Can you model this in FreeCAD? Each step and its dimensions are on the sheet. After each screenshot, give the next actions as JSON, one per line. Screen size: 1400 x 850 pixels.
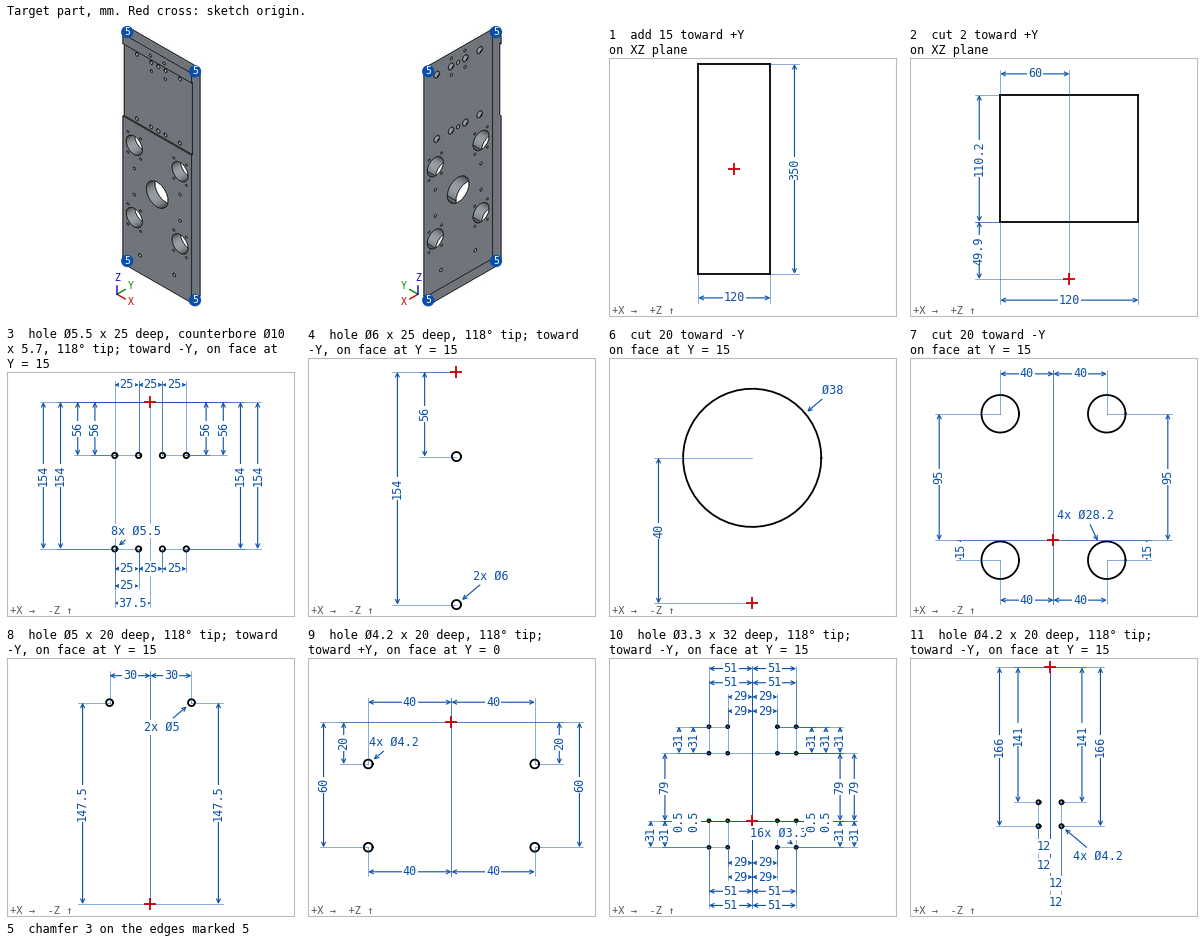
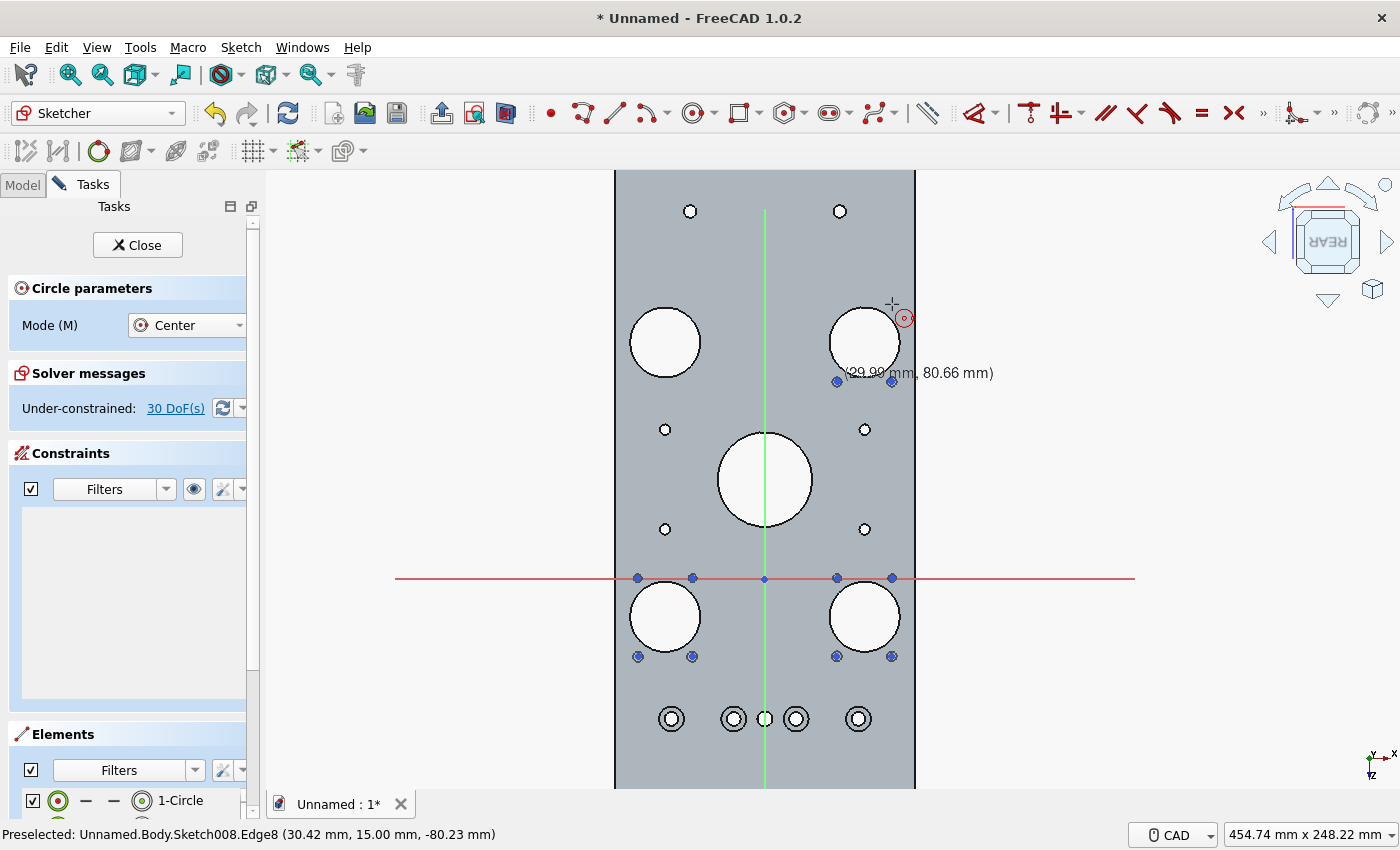
{"action": "left_click", "coordinate": [892, 304]}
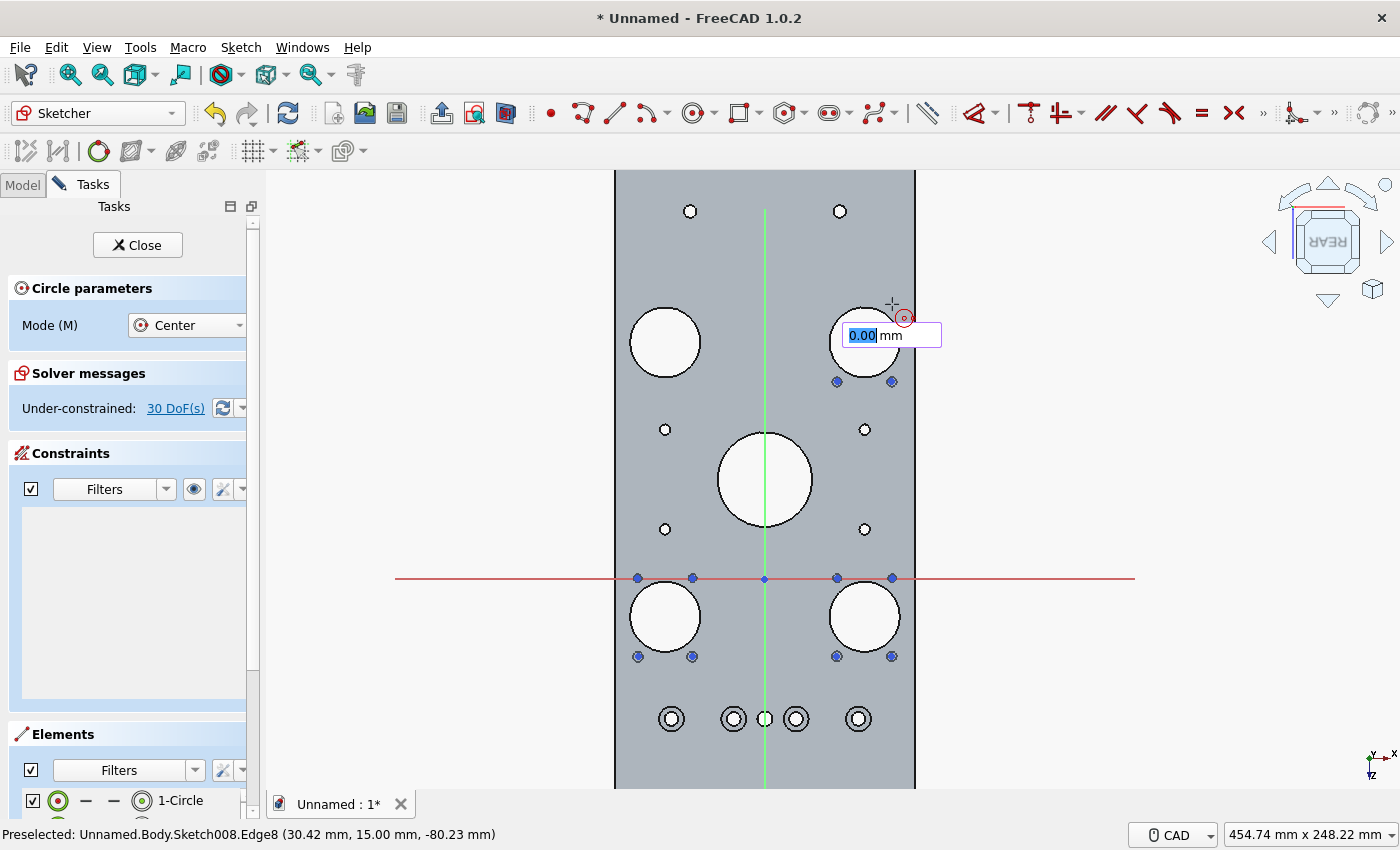
{"action": "scroll", "coordinate": [895, 301], "scroll_direction": "up", "scroll_amount": 7}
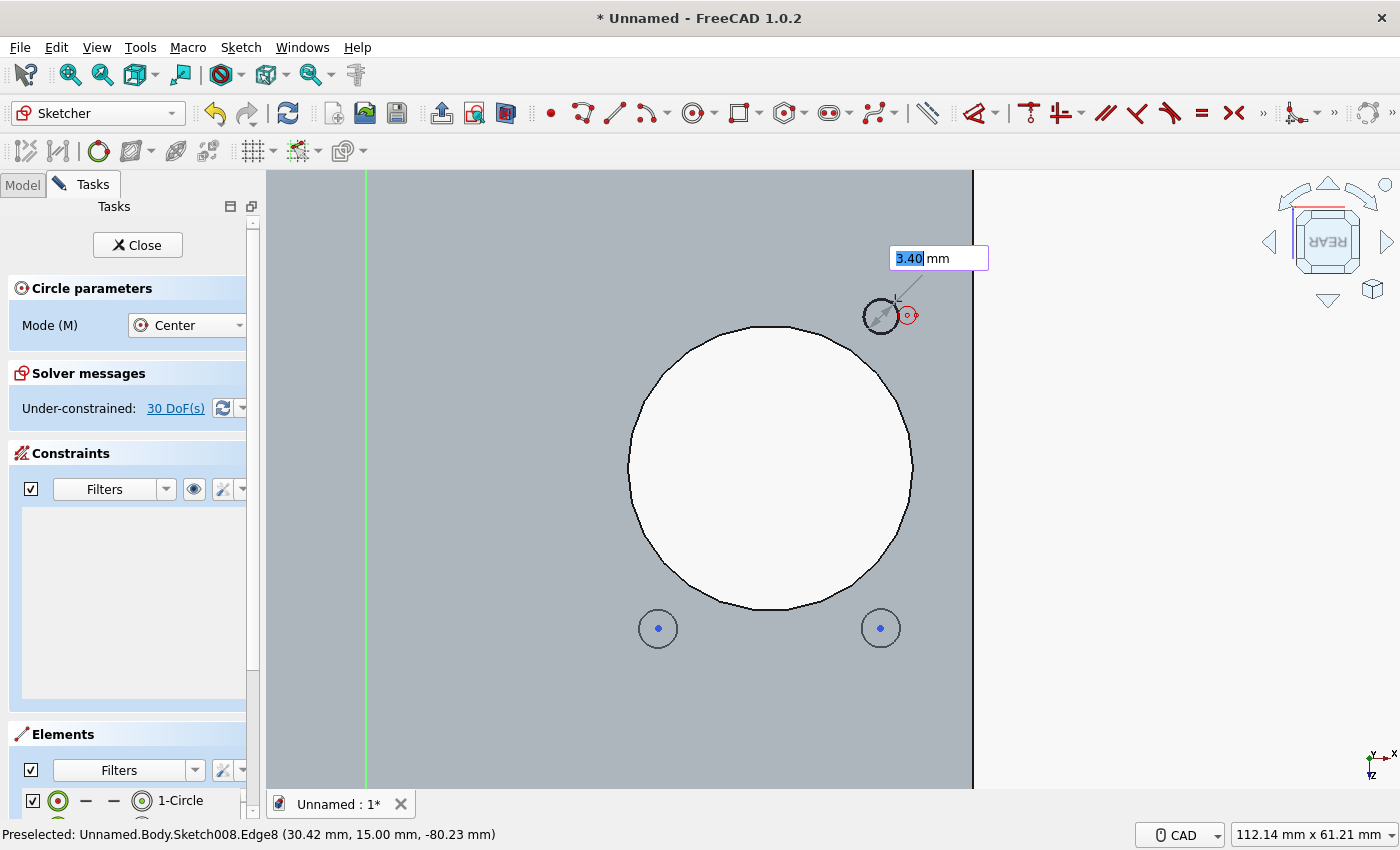
{"action": "left_click", "coordinate": [893, 300]}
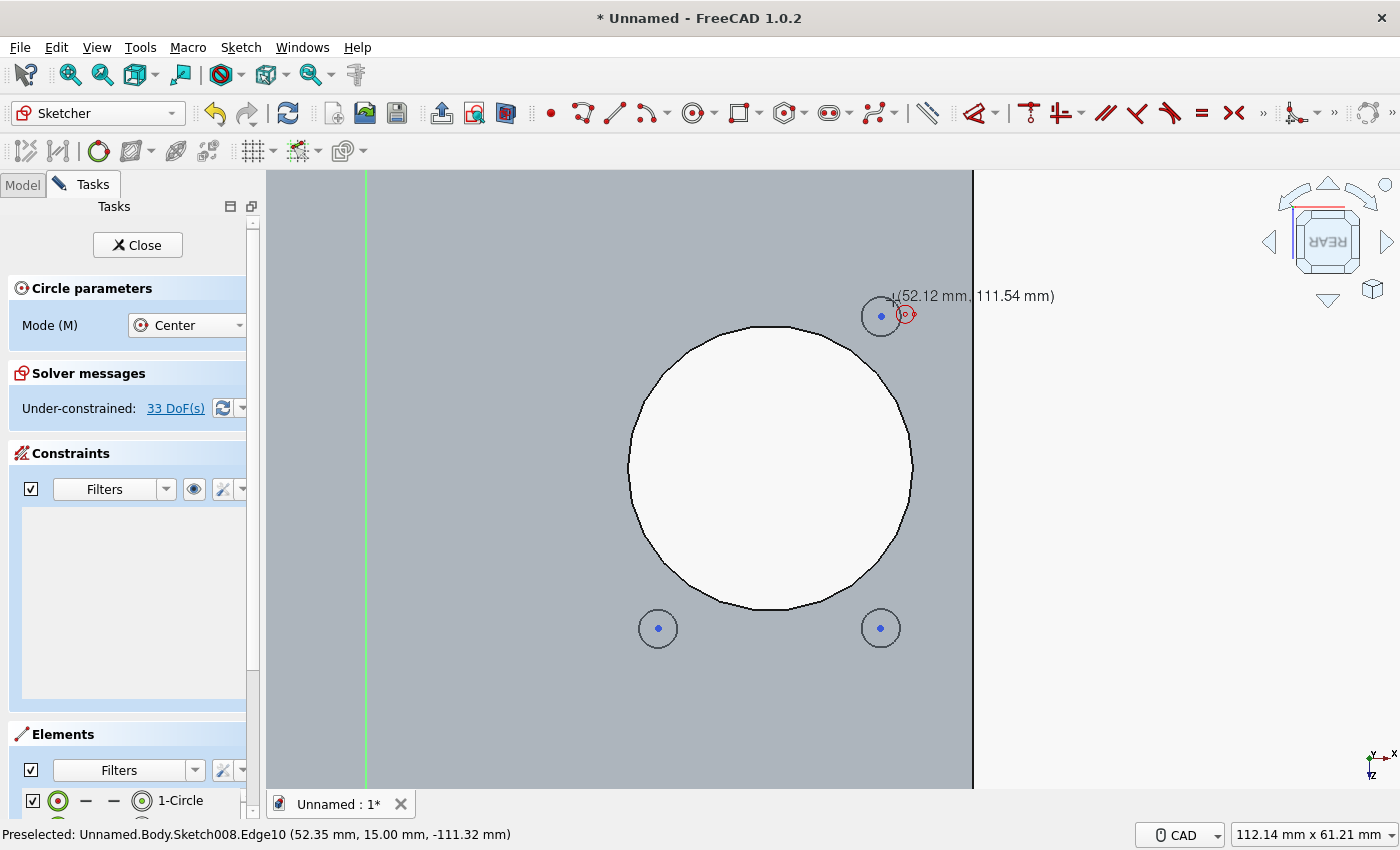
{"action": "scroll", "coordinate": [659, 312], "scroll_direction": "up", "scroll_amount": 2}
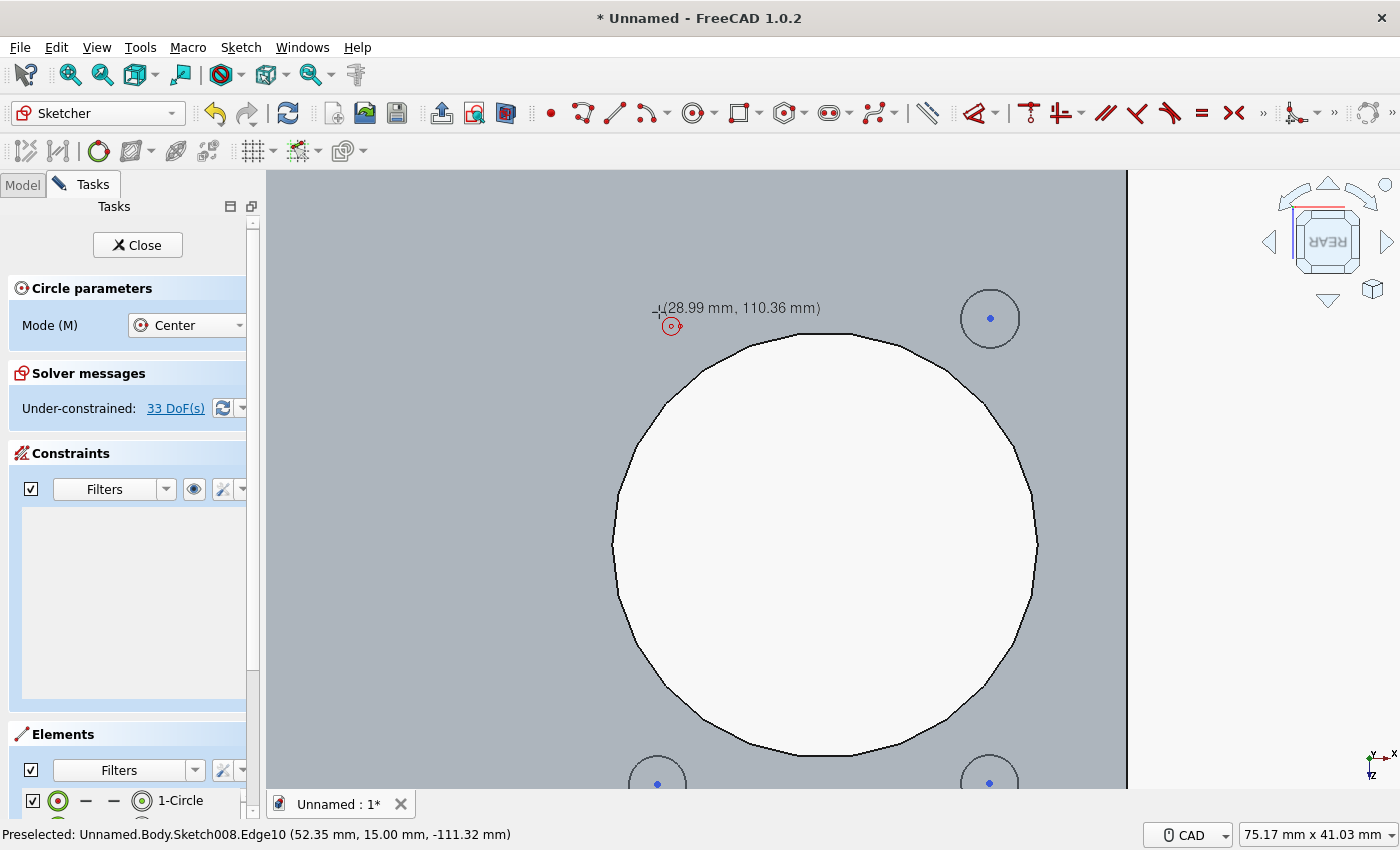
{"action": "scroll", "coordinate": [872, 302], "scroll_direction": "down", "scroll_amount": 9}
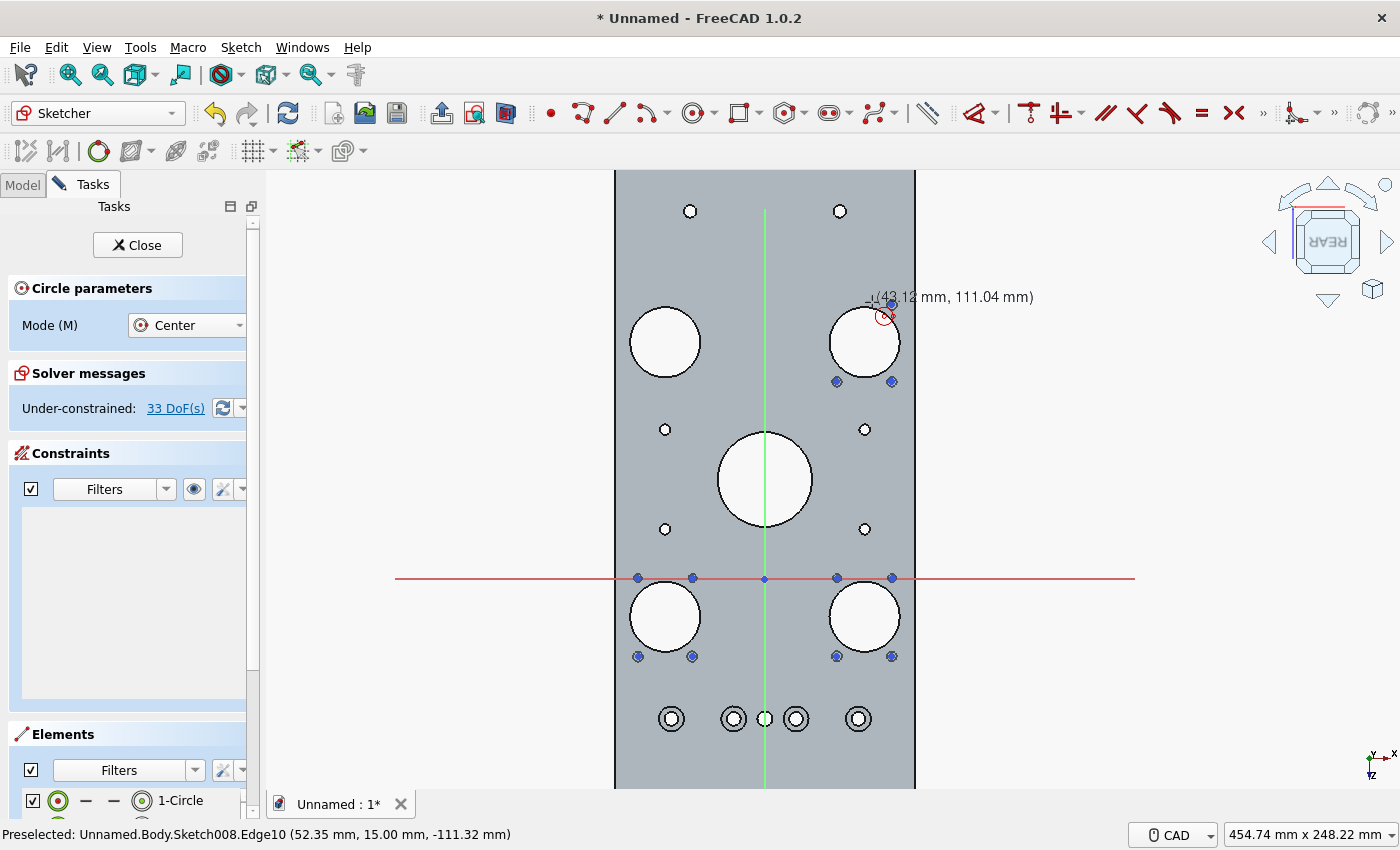
{"action": "left_click", "coordinate": [837, 304]}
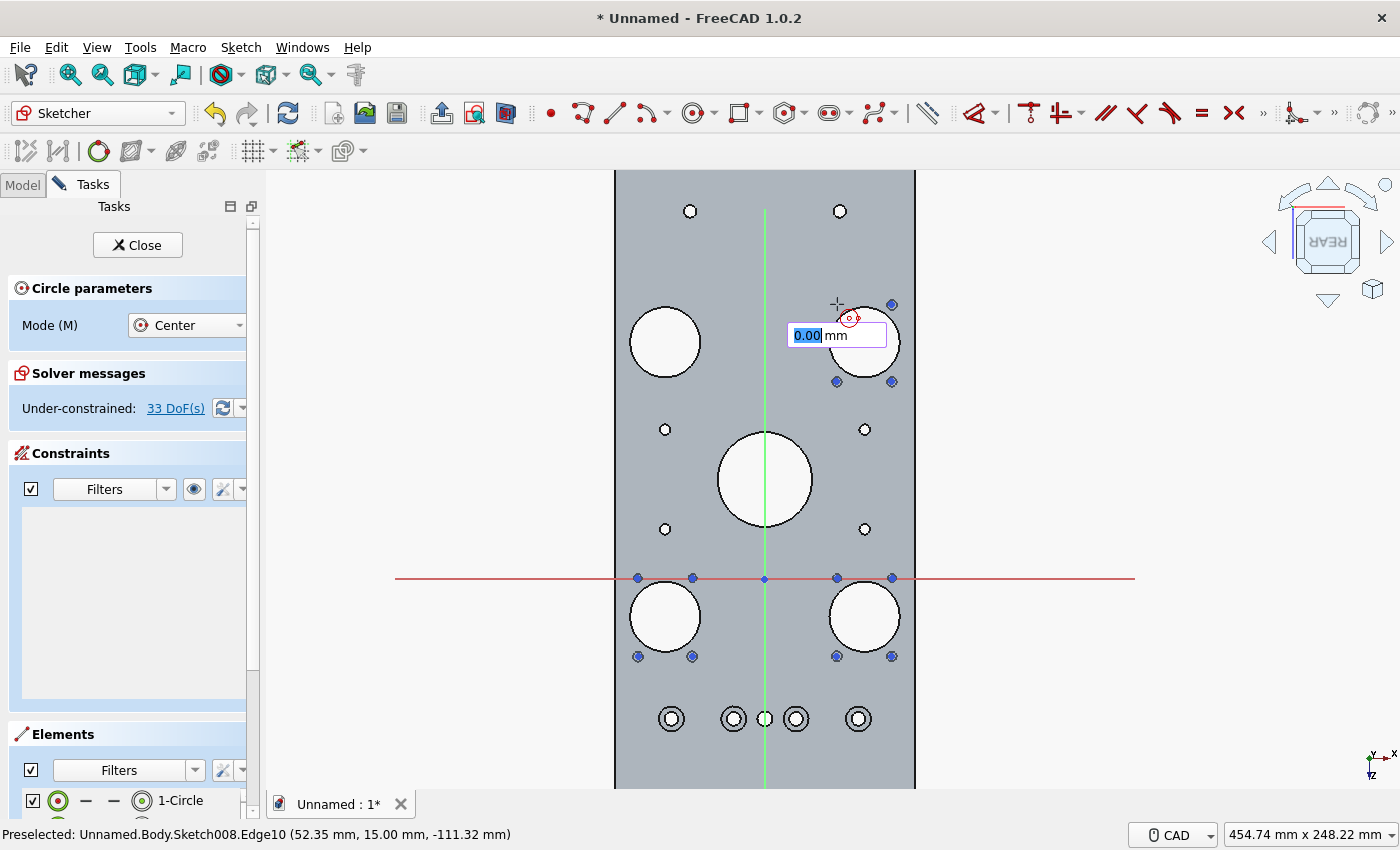
{"action": "scroll", "coordinate": [840, 301], "scroll_direction": "up", "scroll_amount": 7}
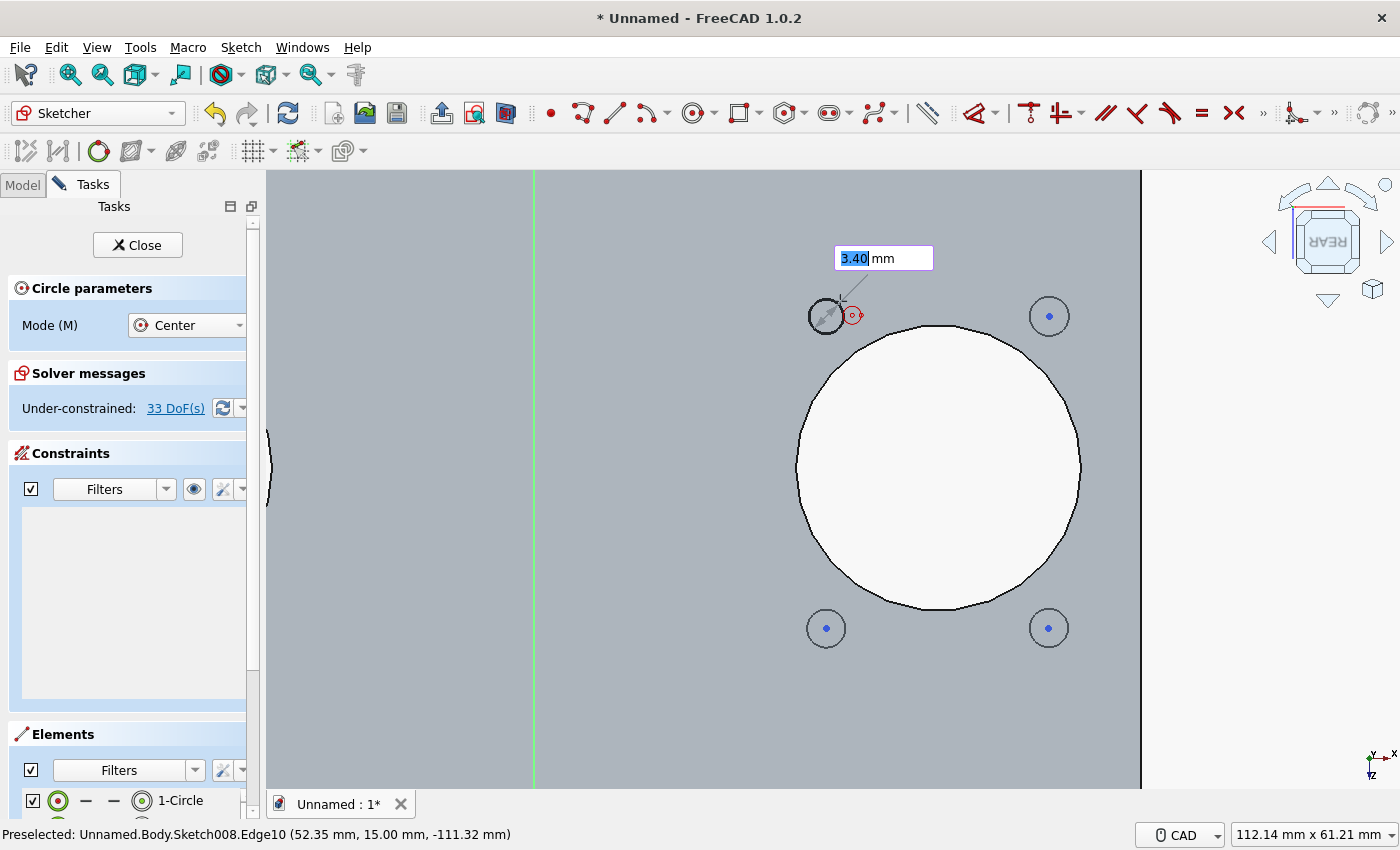
{"action": "left_click", "coordinate": [839, 299]}